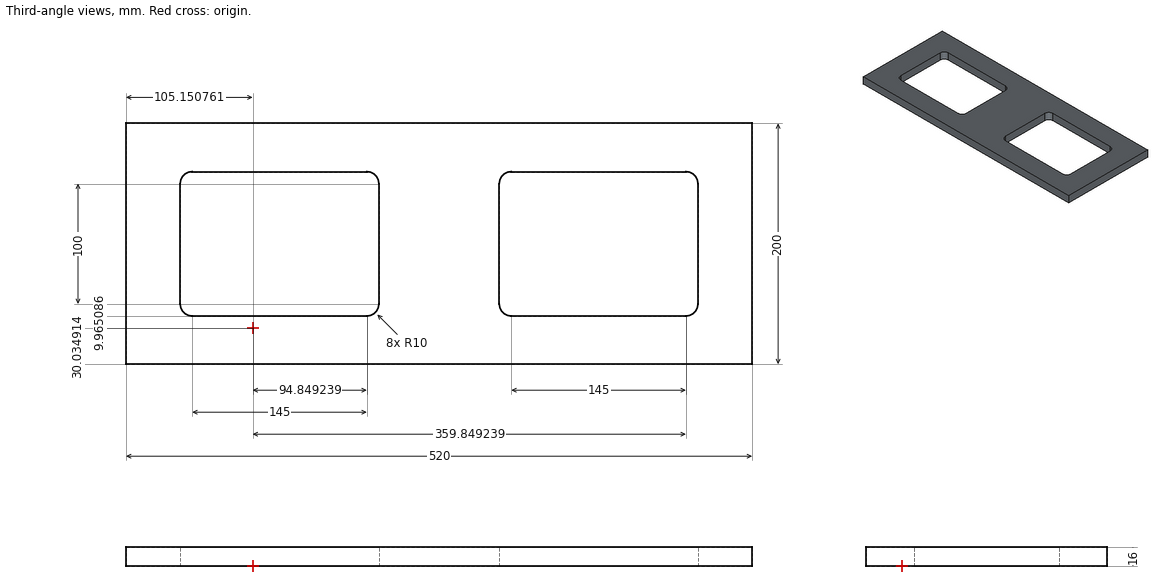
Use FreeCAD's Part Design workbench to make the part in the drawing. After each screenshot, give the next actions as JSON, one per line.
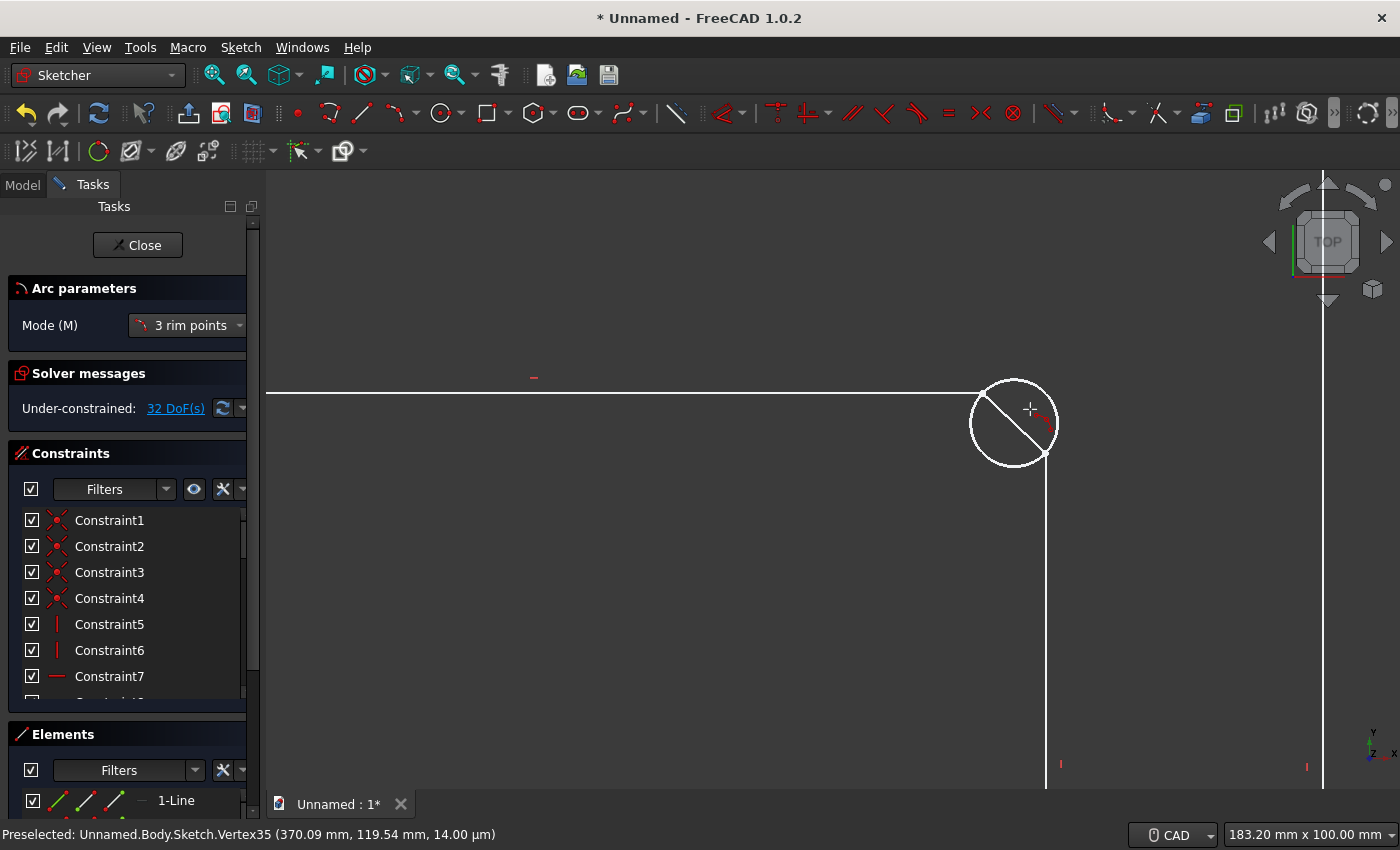
{"action": "left_click", "coordinate": [1026, 407]}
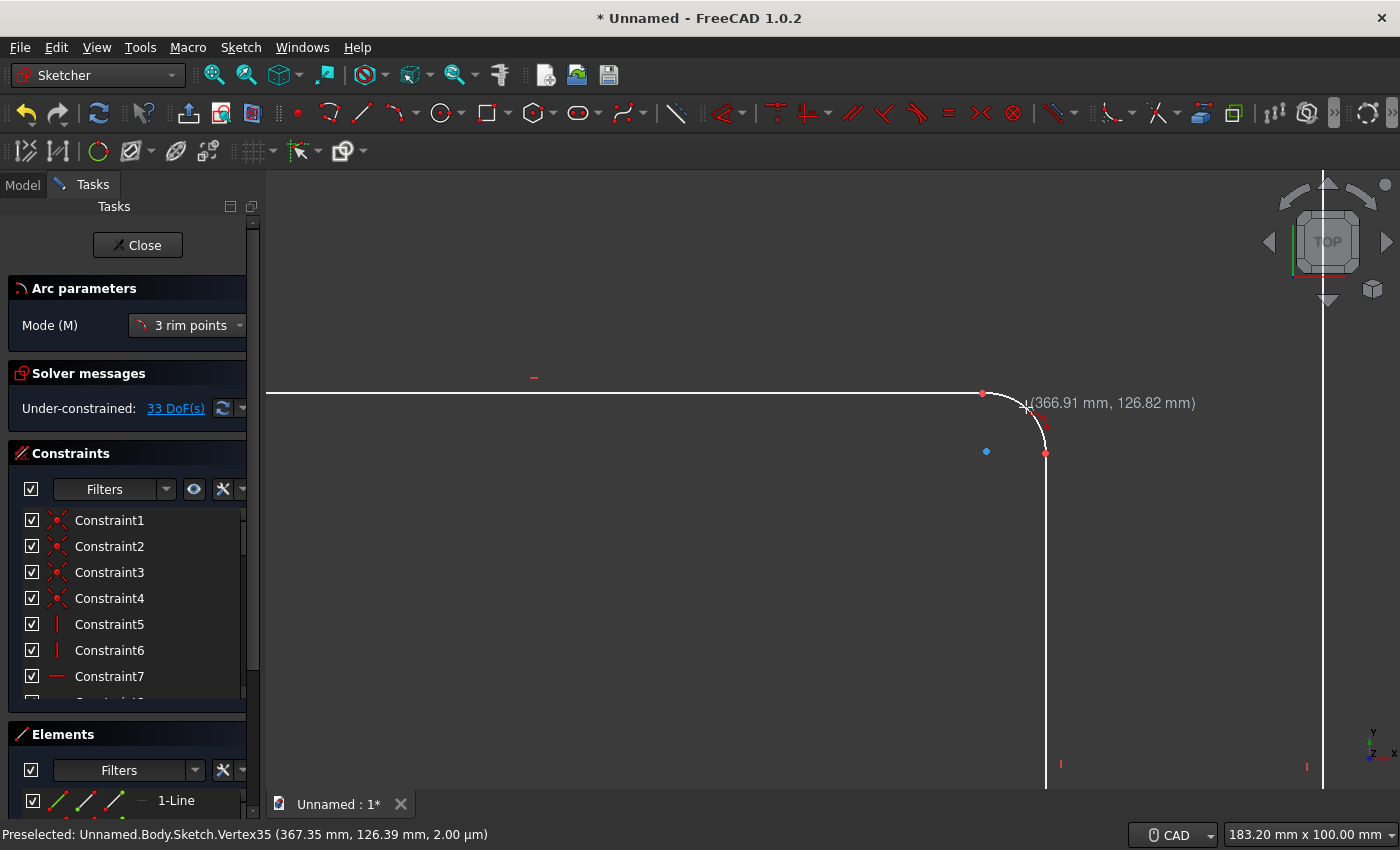
{"action": "scroll", "coordinate": [1030, 409], "scroll_direction": "down", "scroll_amount": 8}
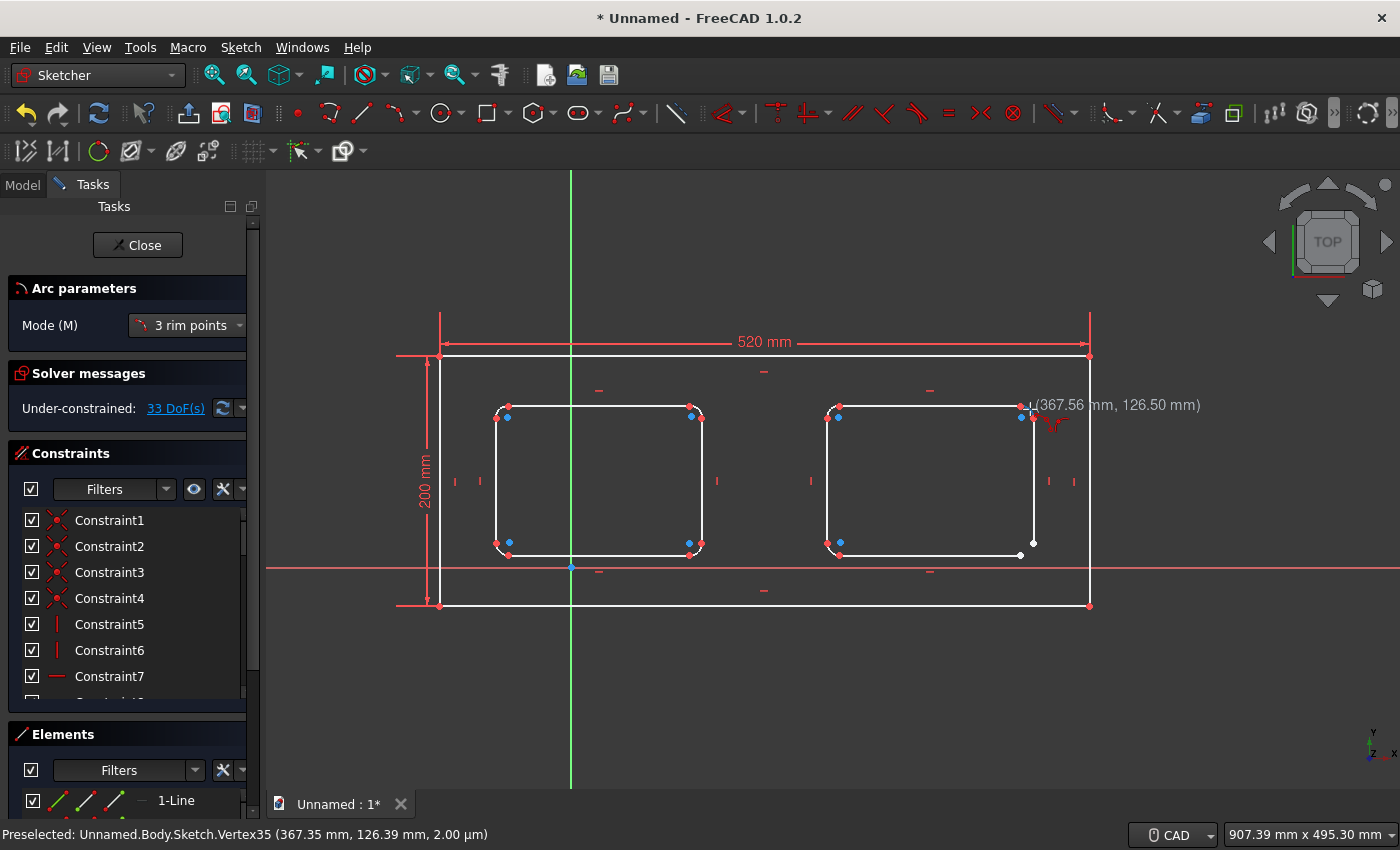
{"action": "left_click", "coordinate": [1034, 544]}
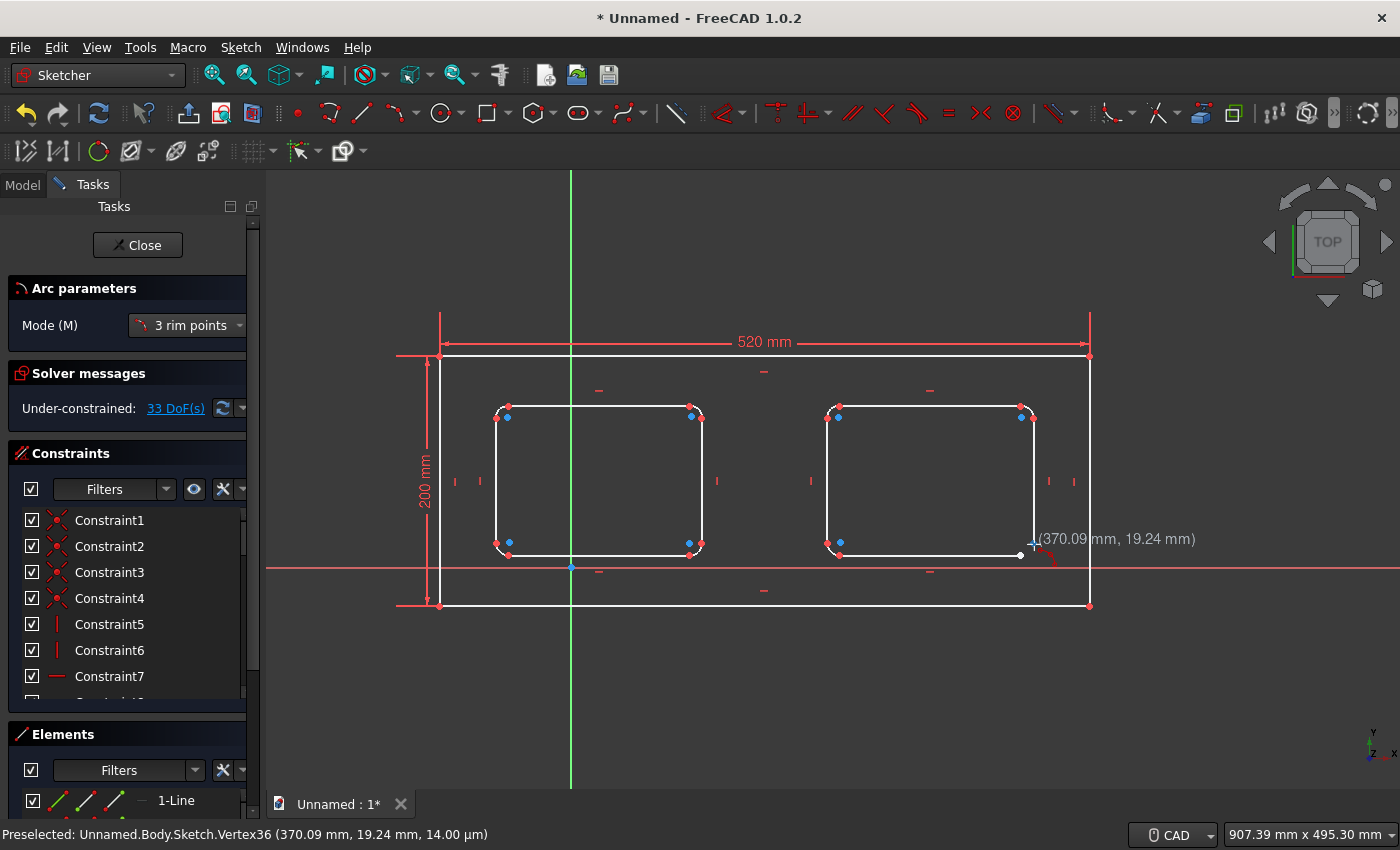
{"action": "scroll", "coordinate": [1021, 555], "scroll_direction": "up", "scroll_amount": 2}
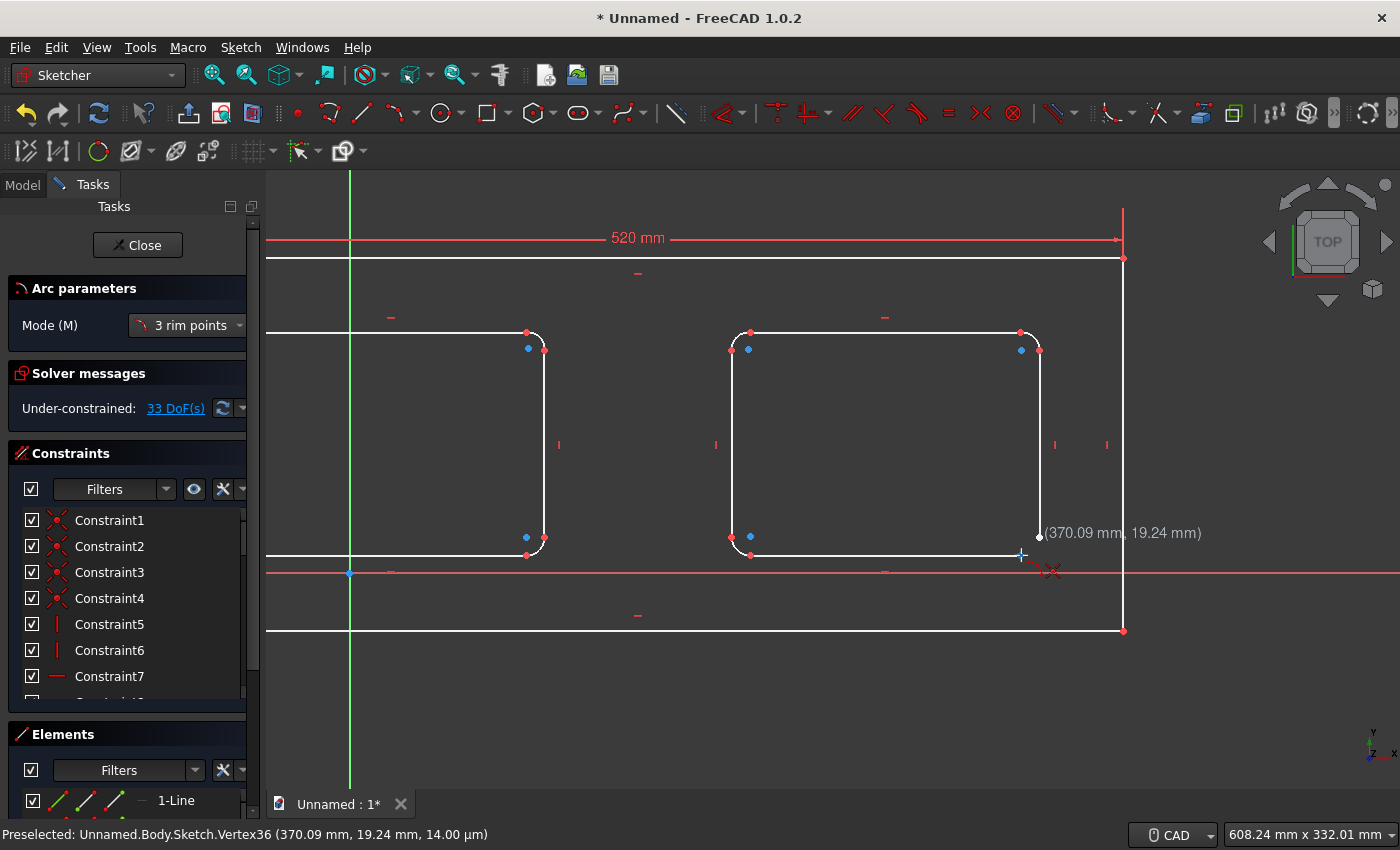
{"action": "left_click", "coordinate": [1021, 556]}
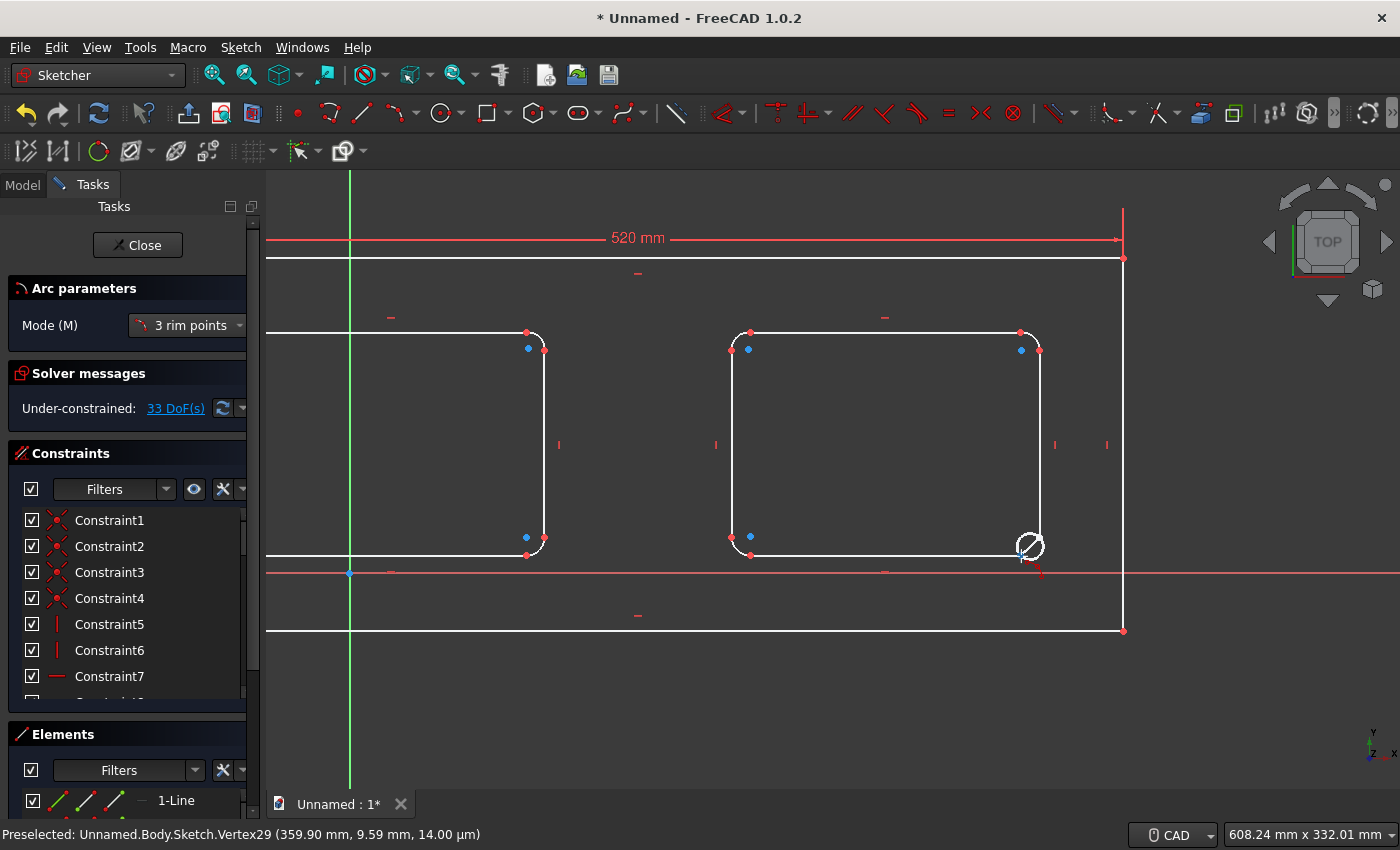
{"action": "scroll", "coordinate": [1034, 549], "scroll_direction": "up", "scroll_amount": 6}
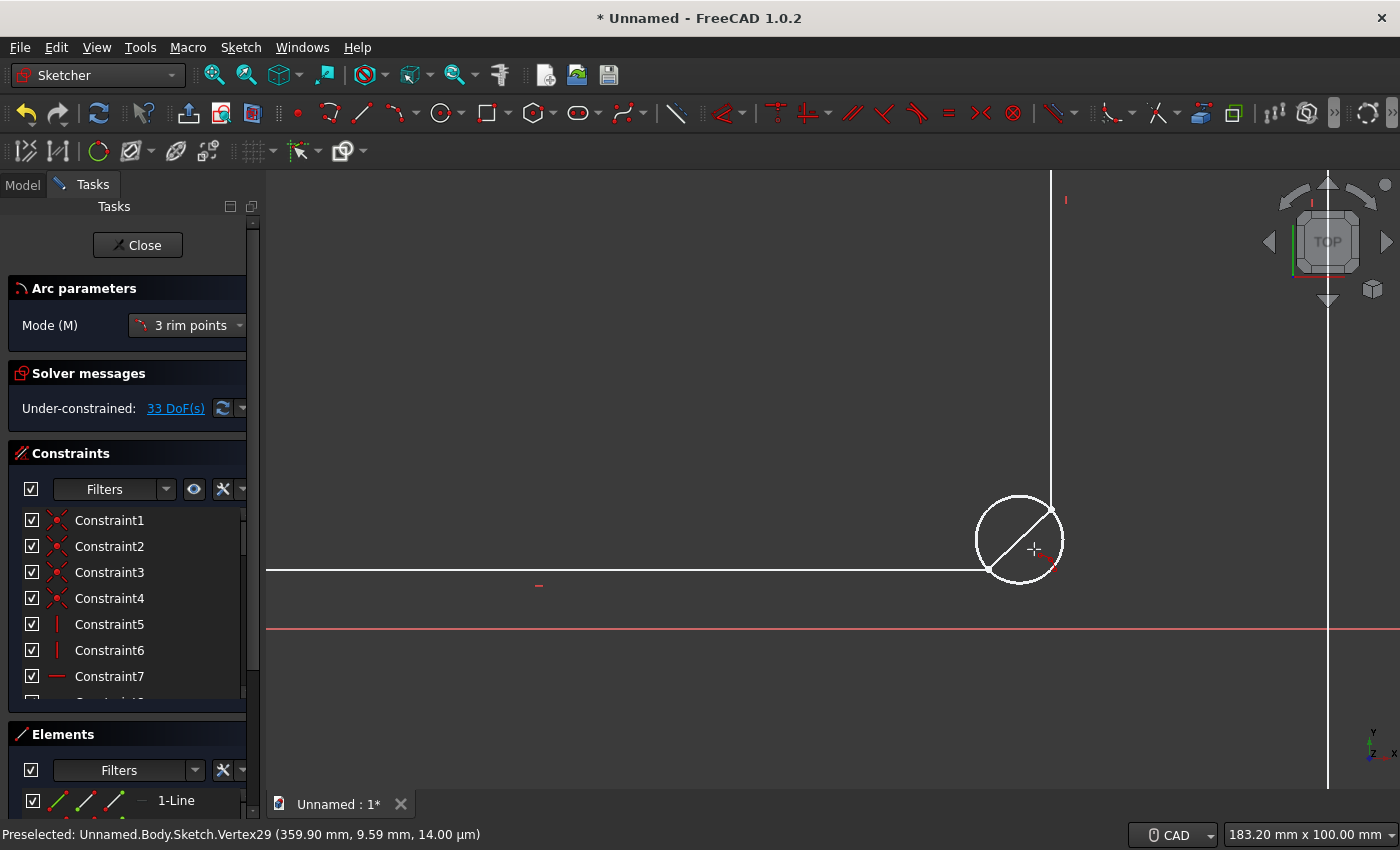
{"action": "left_click", "coordinate": [1031, 549]}
{"action": "key", "text": "Escape"}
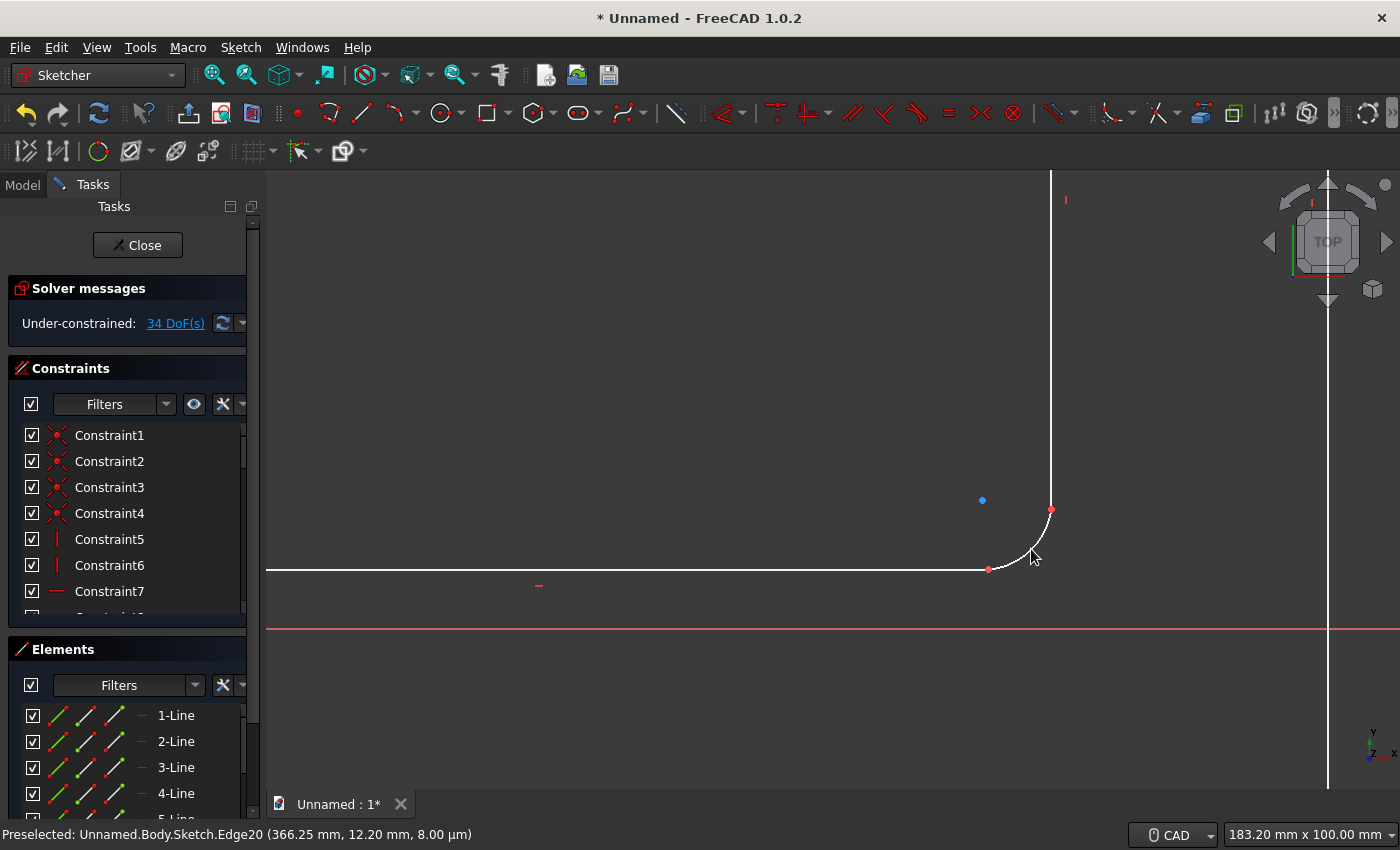
{"action": "scroll", "coordinate": [1029, 551], "scroll_direction": "down", "scroll_amount": 8}